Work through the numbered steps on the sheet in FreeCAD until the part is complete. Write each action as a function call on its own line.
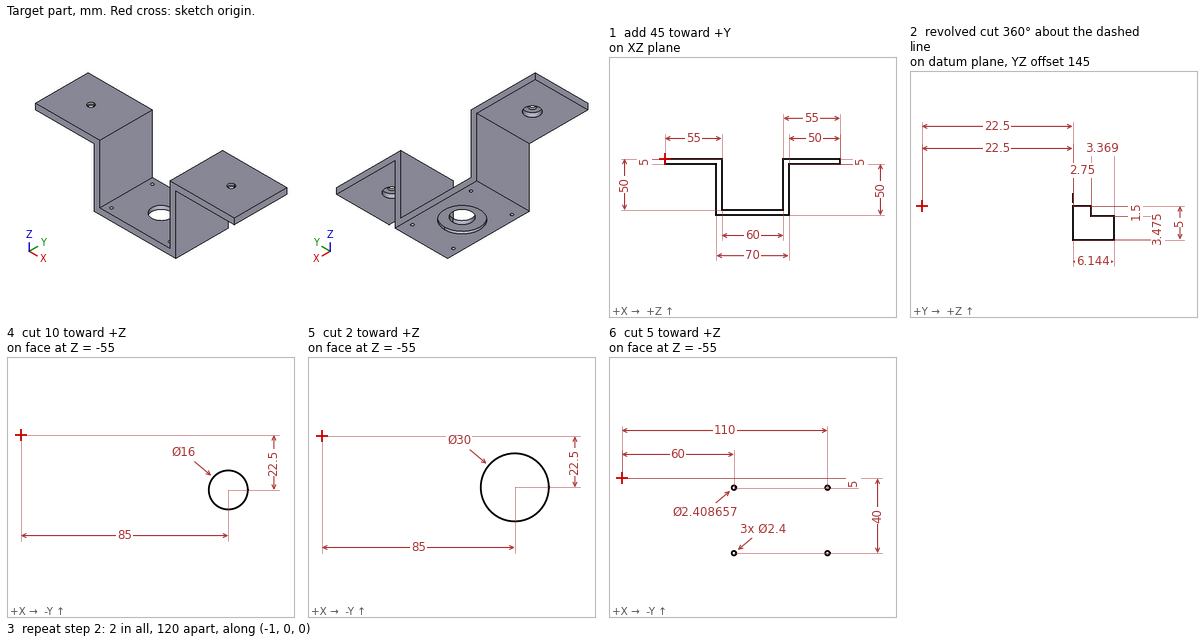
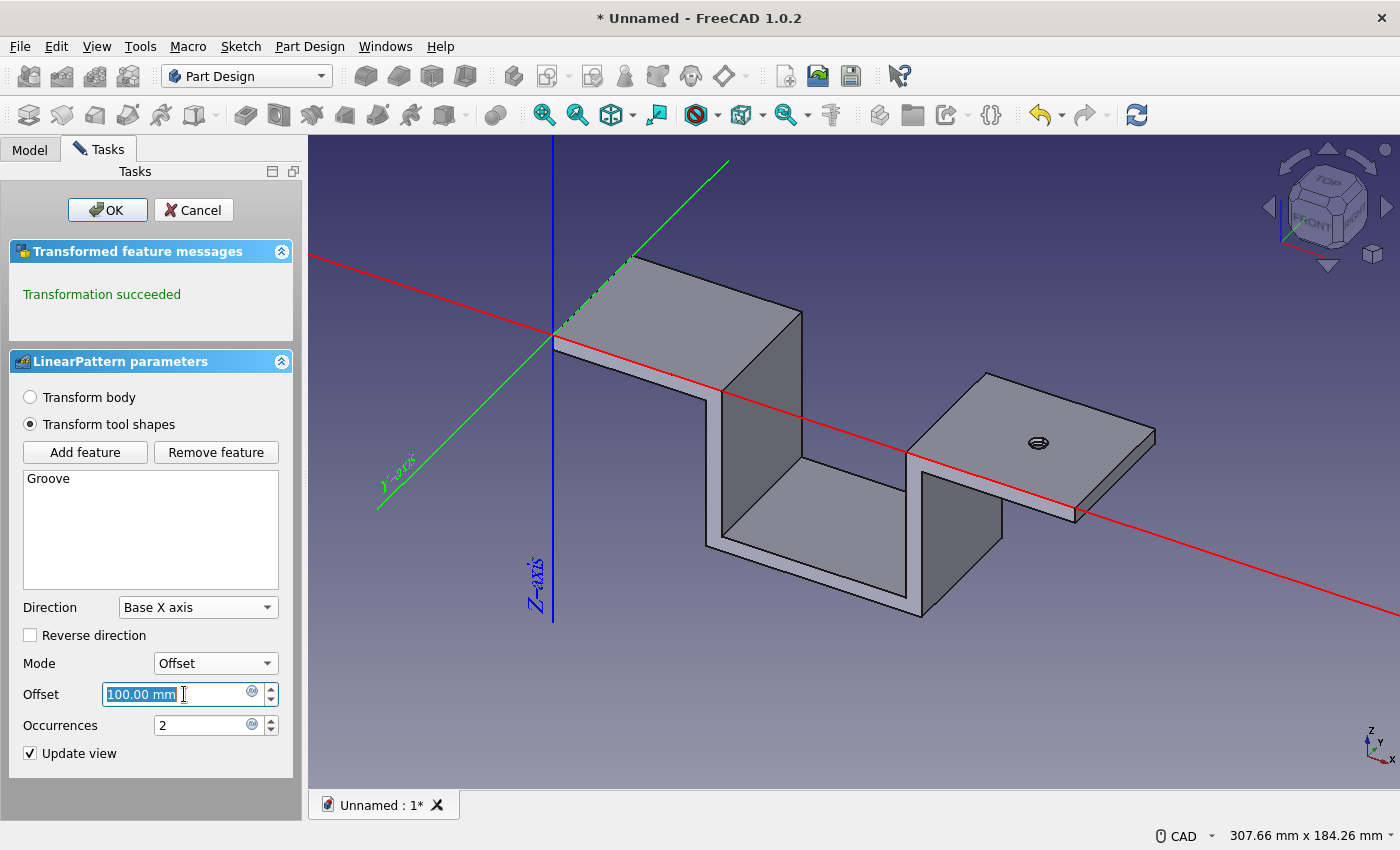
text(120)
key(Tab)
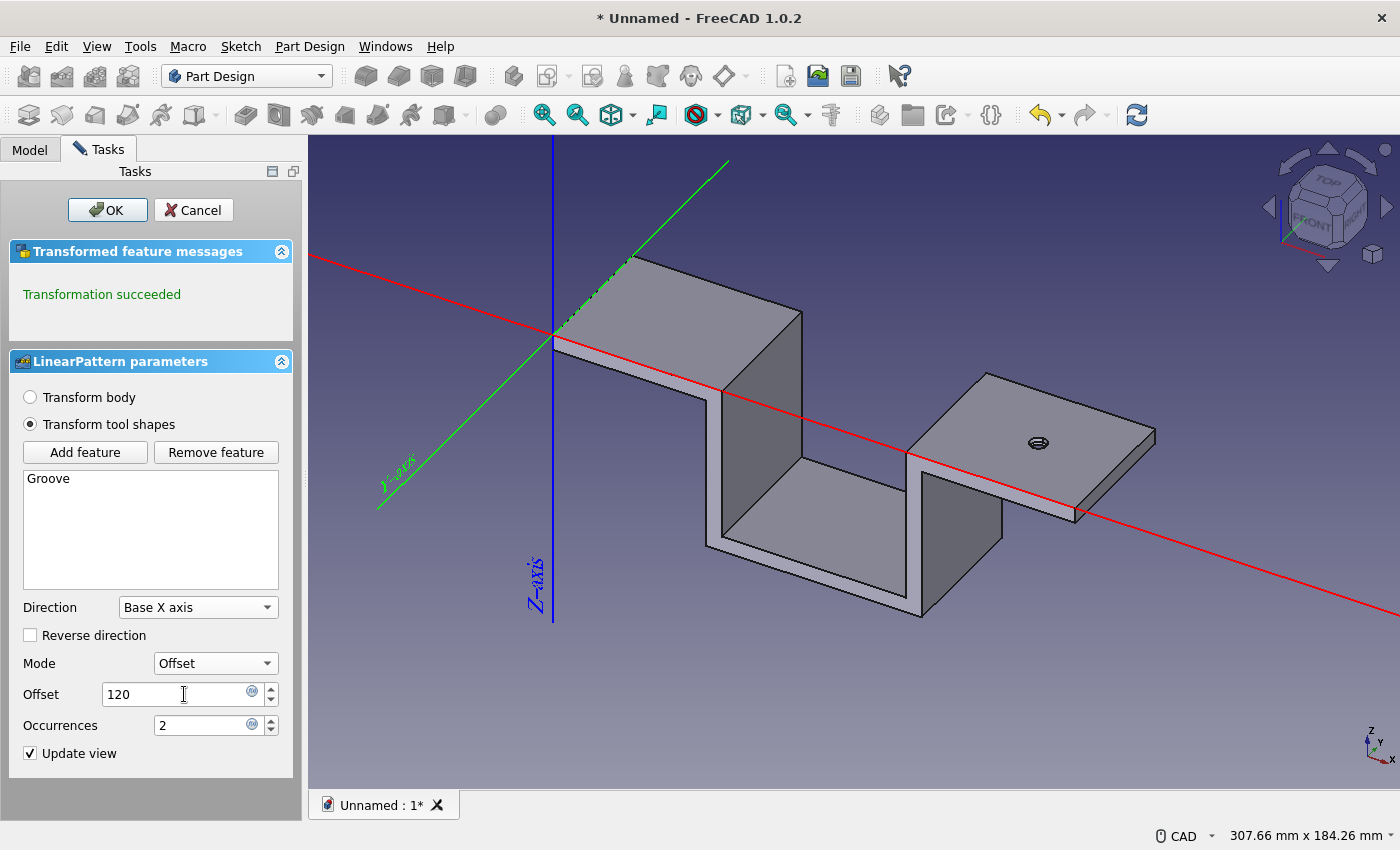
triple_click(210, 726)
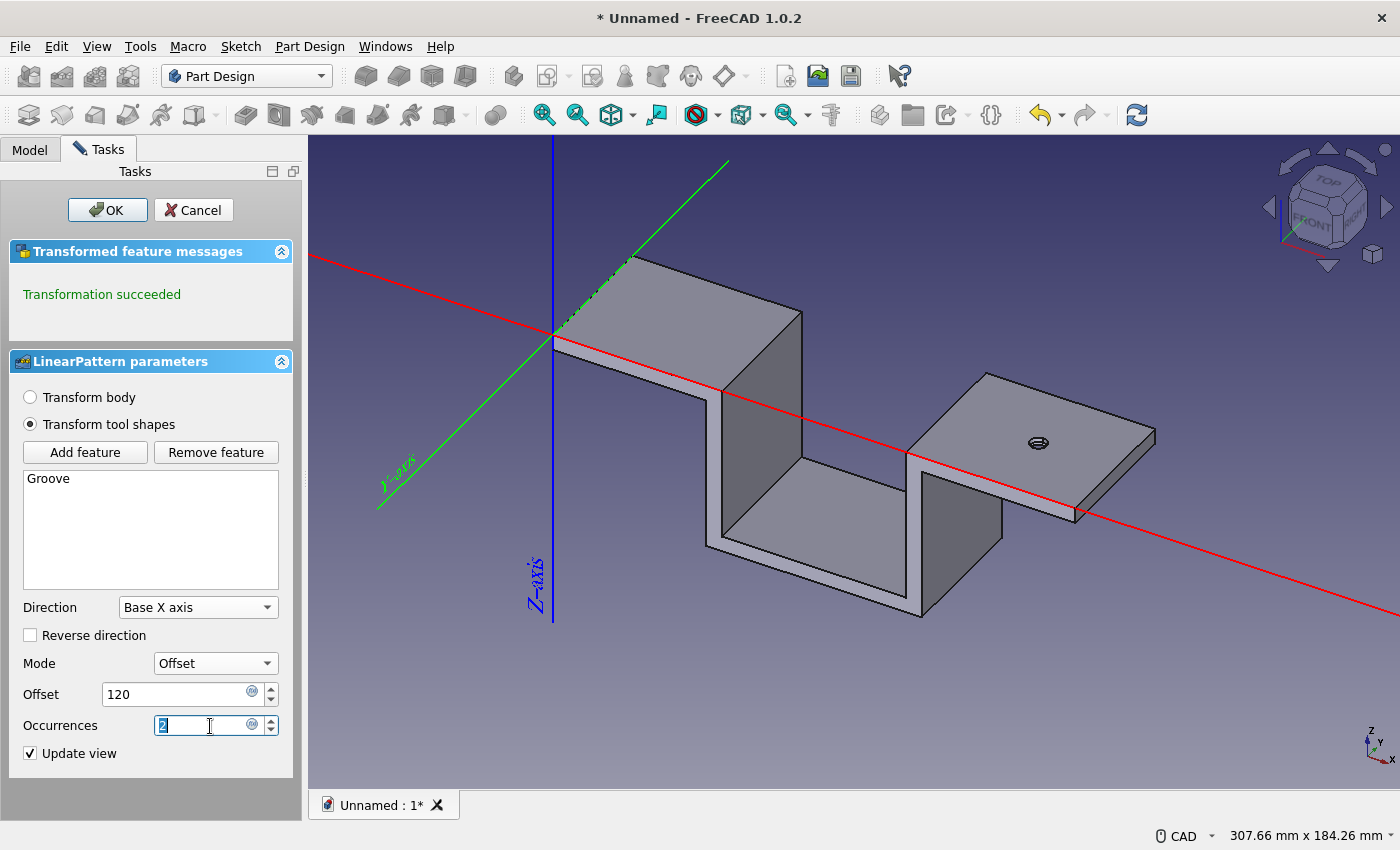
text(2)
key(Tab)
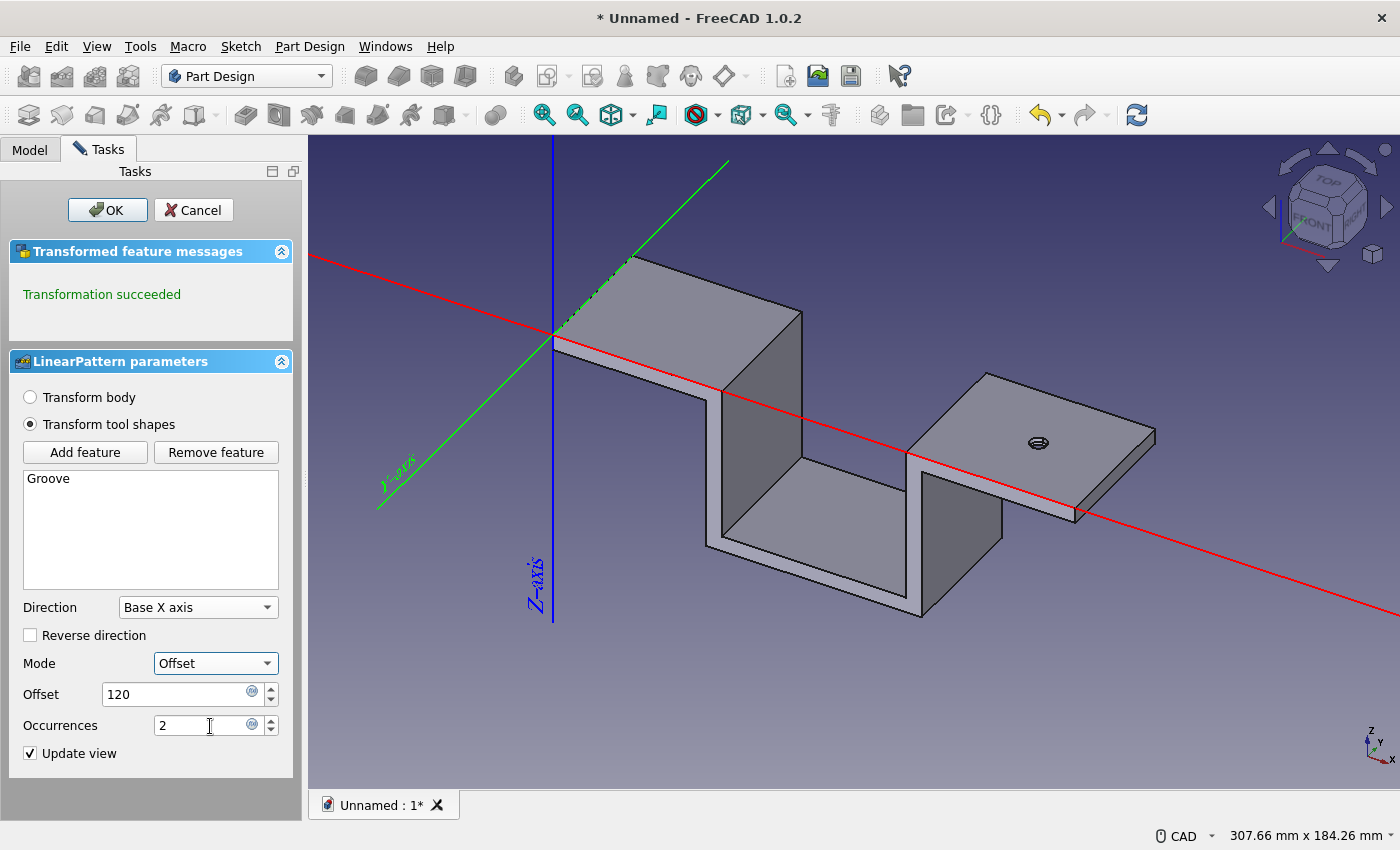
click(31, 635)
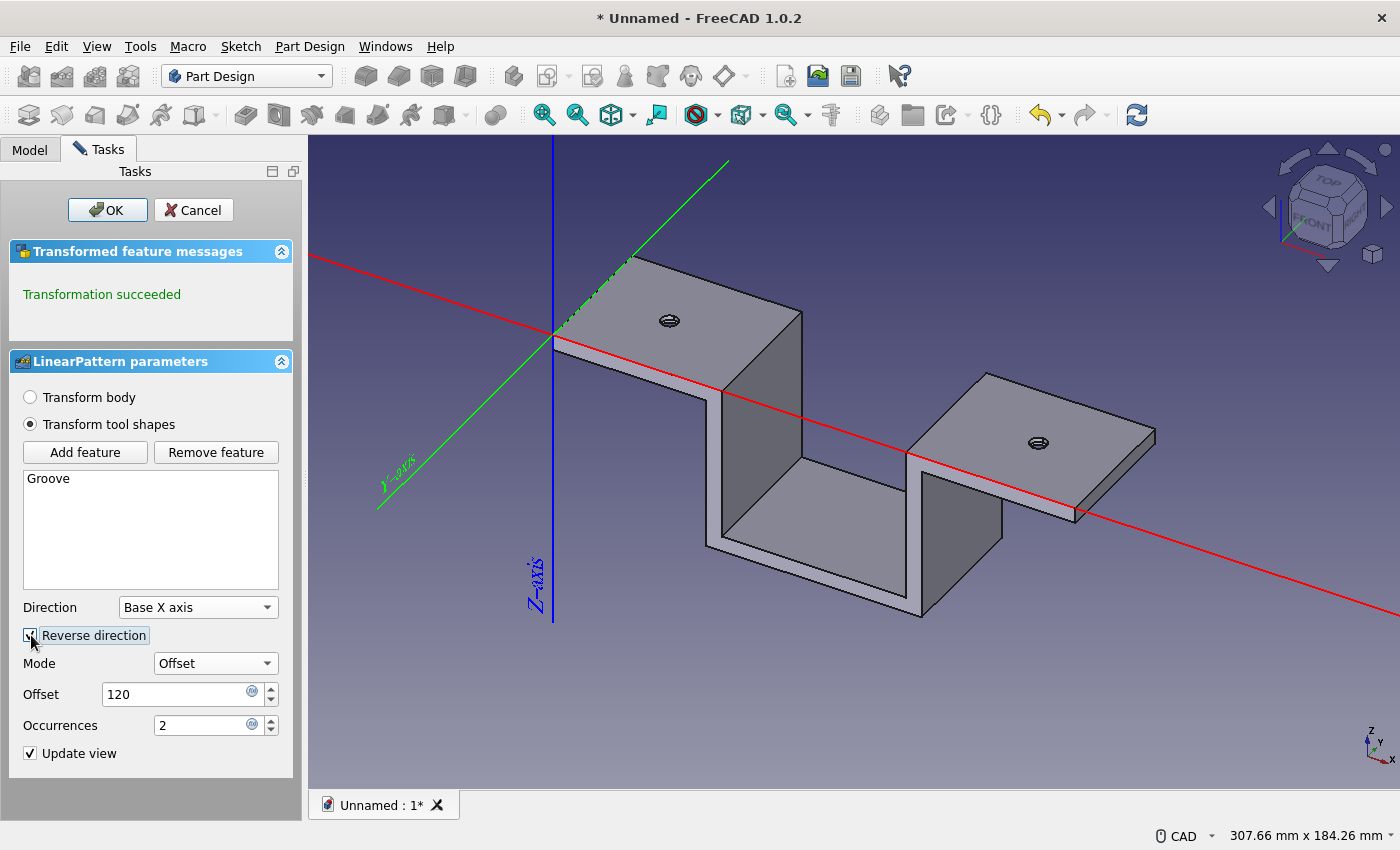
click(108, 210)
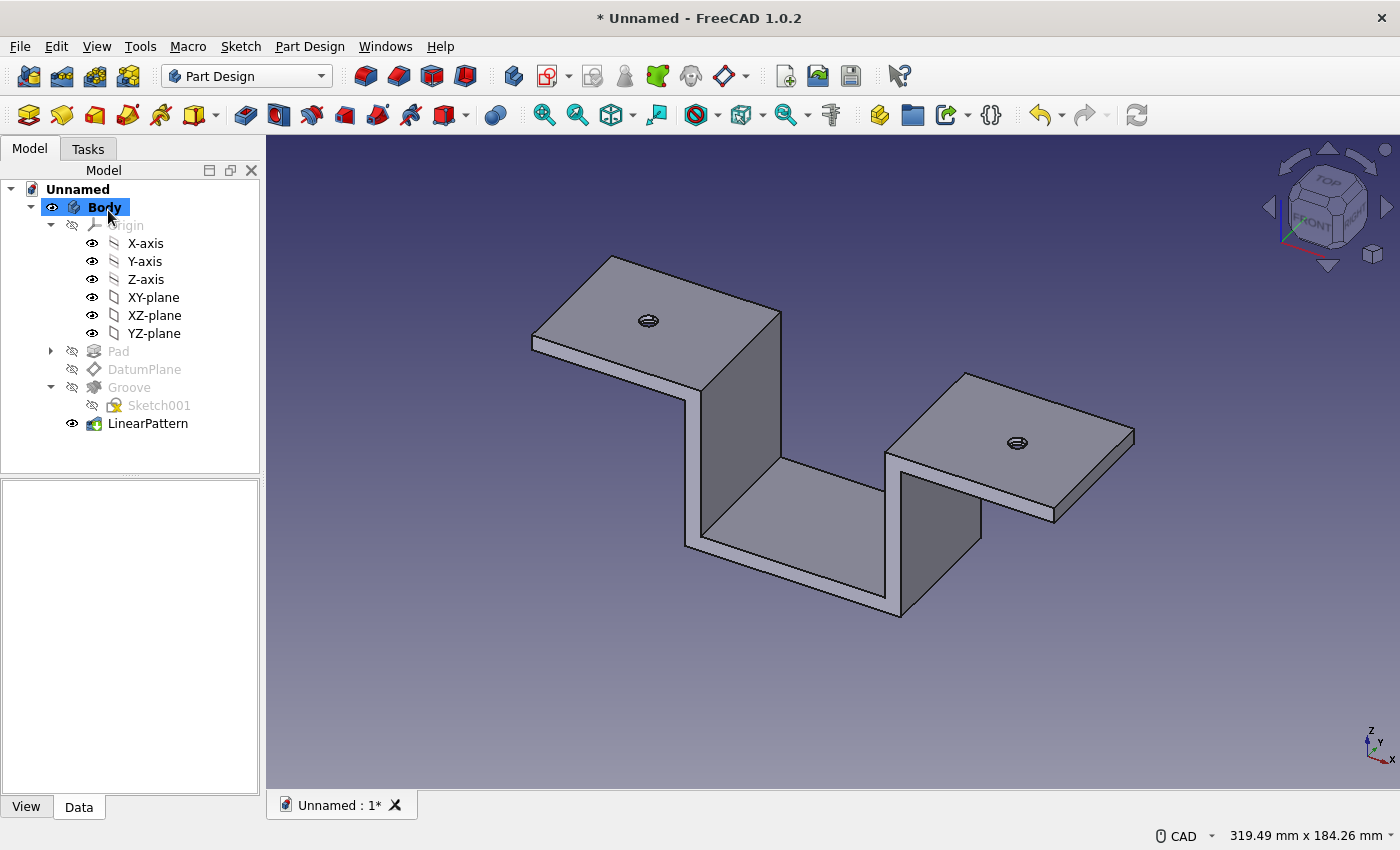
key(5)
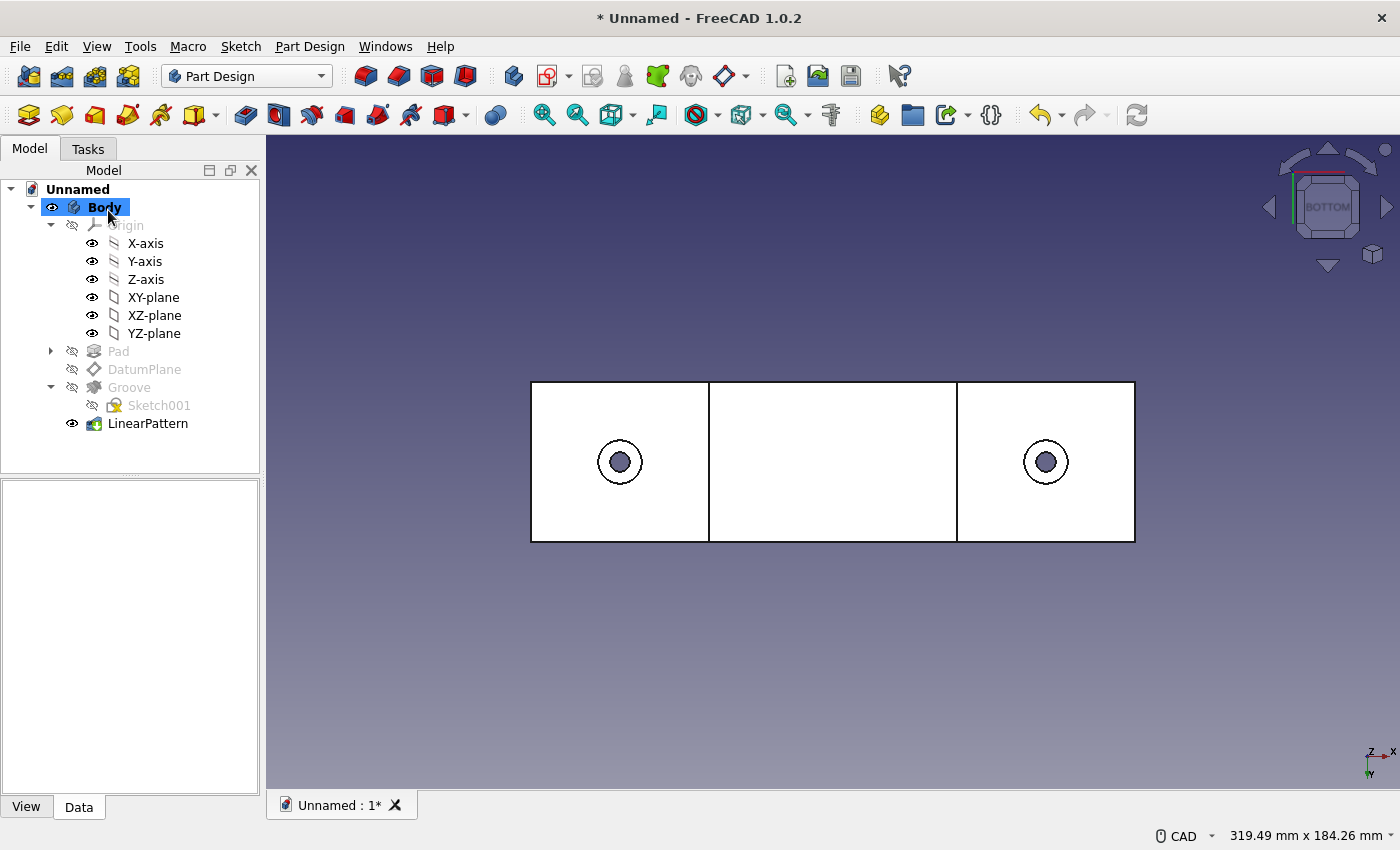
click(868, 461)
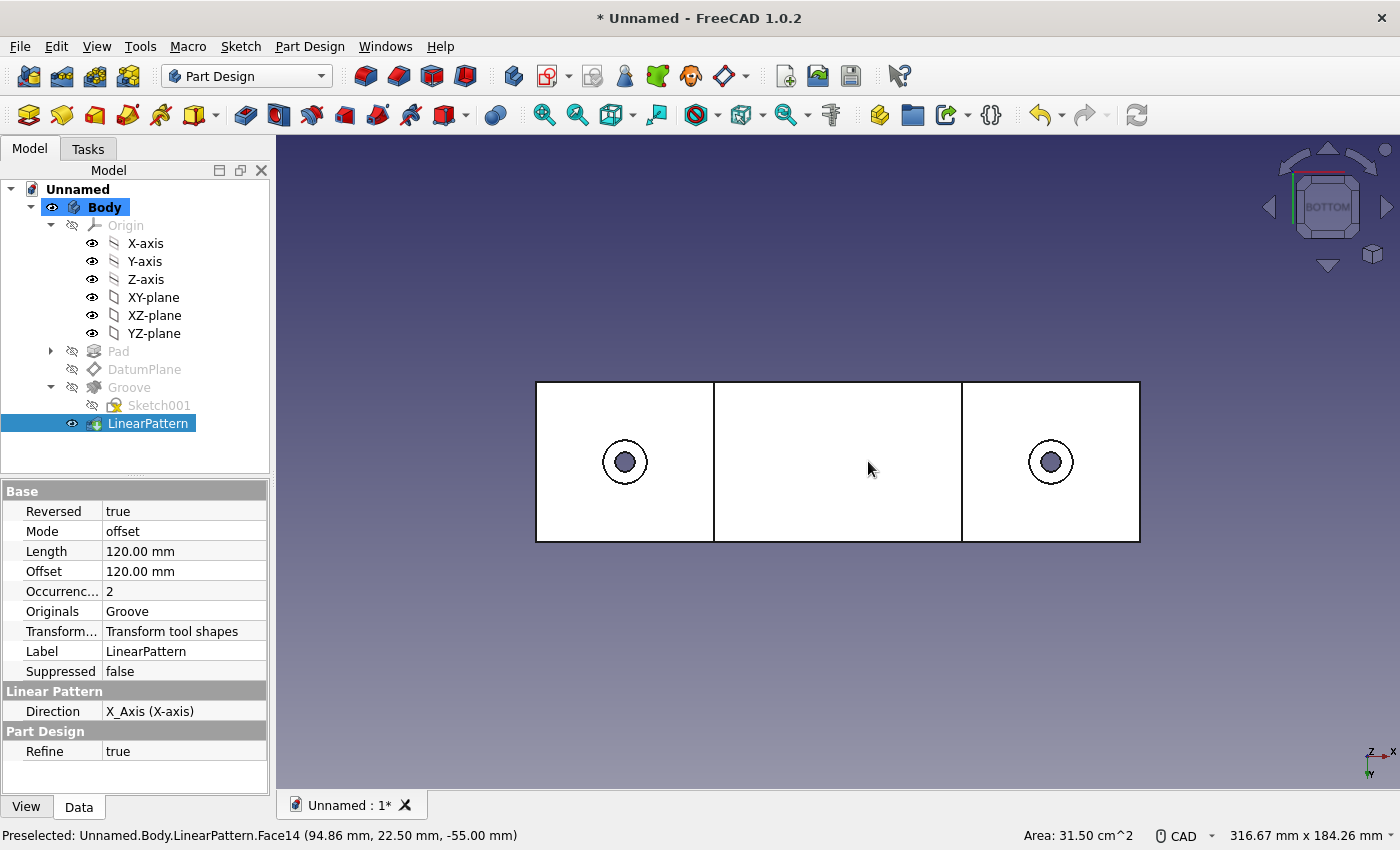
click(546, 76)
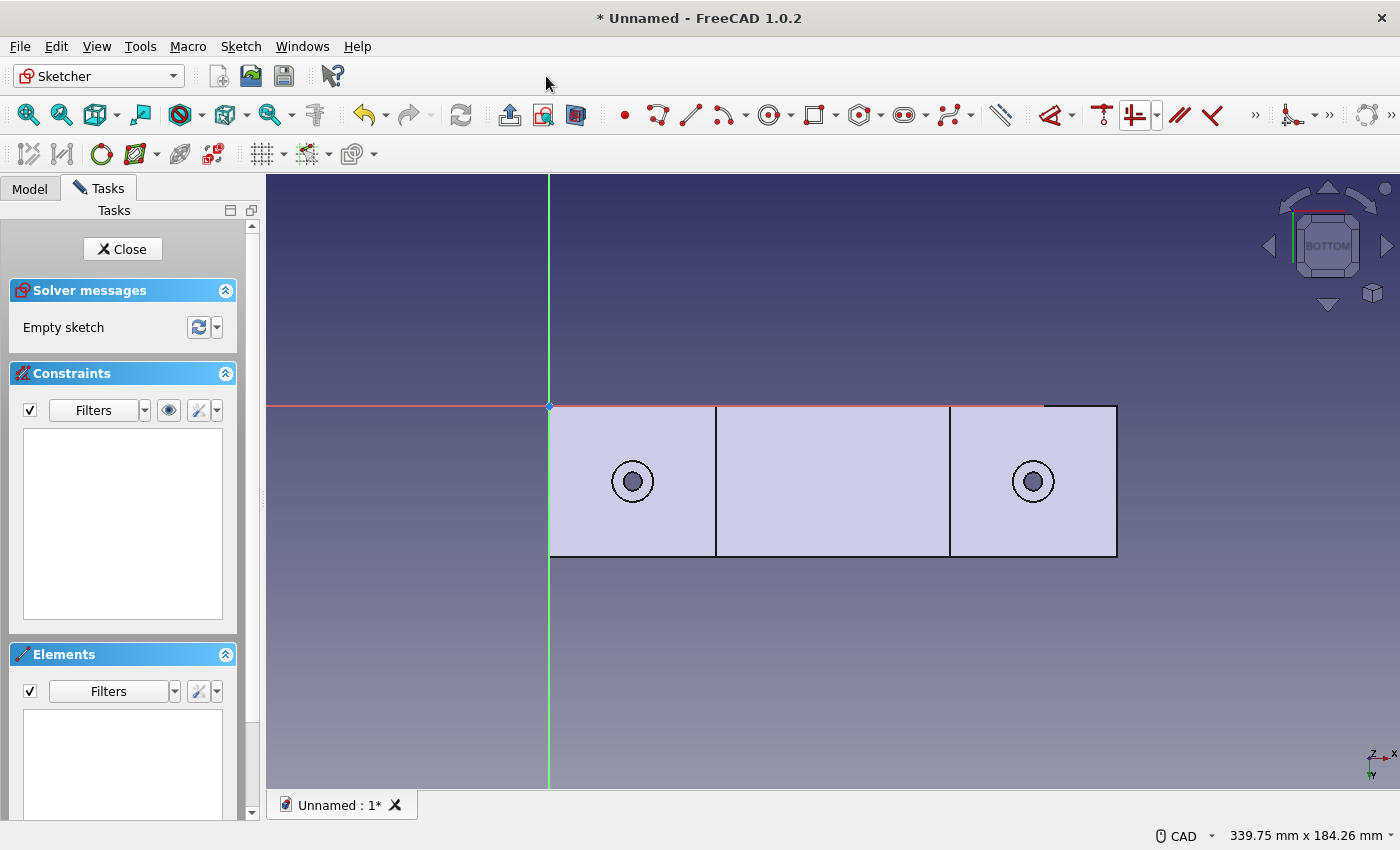
scroll(844, 481, up, 10)